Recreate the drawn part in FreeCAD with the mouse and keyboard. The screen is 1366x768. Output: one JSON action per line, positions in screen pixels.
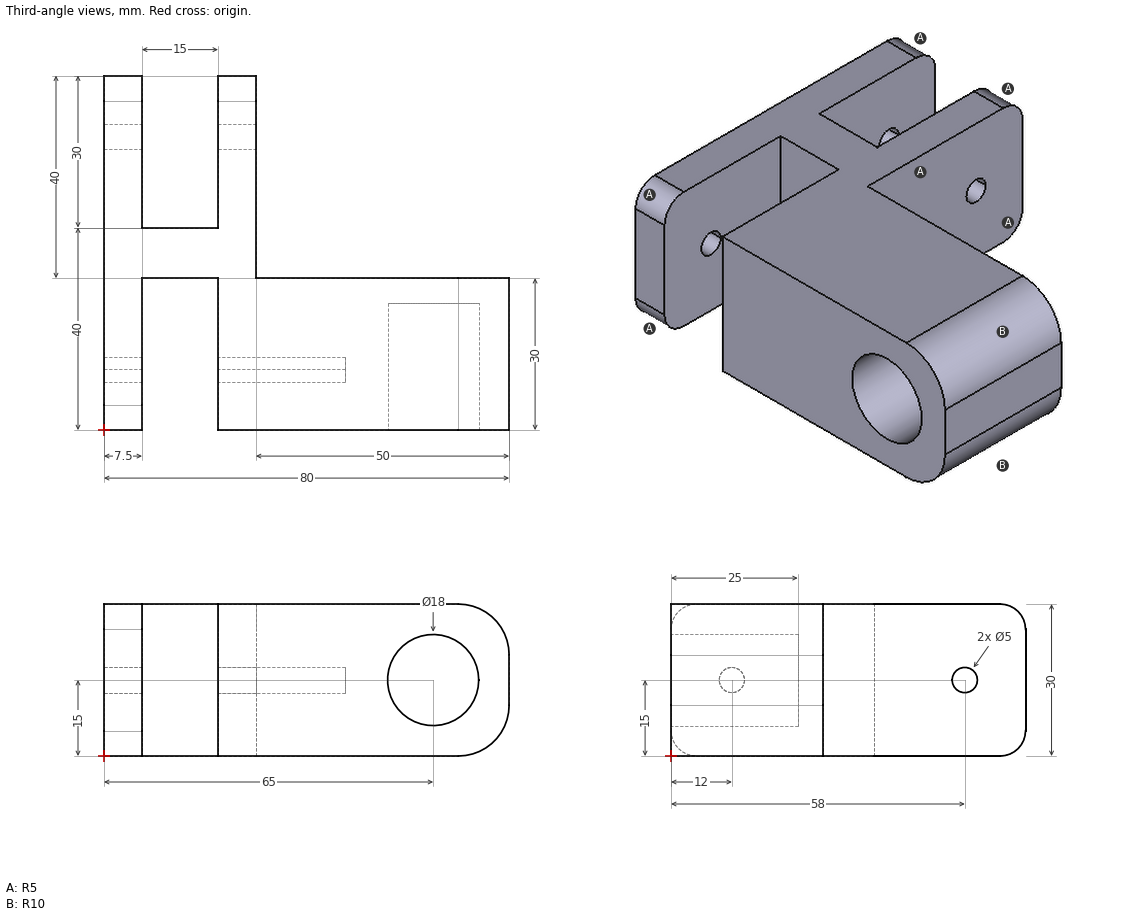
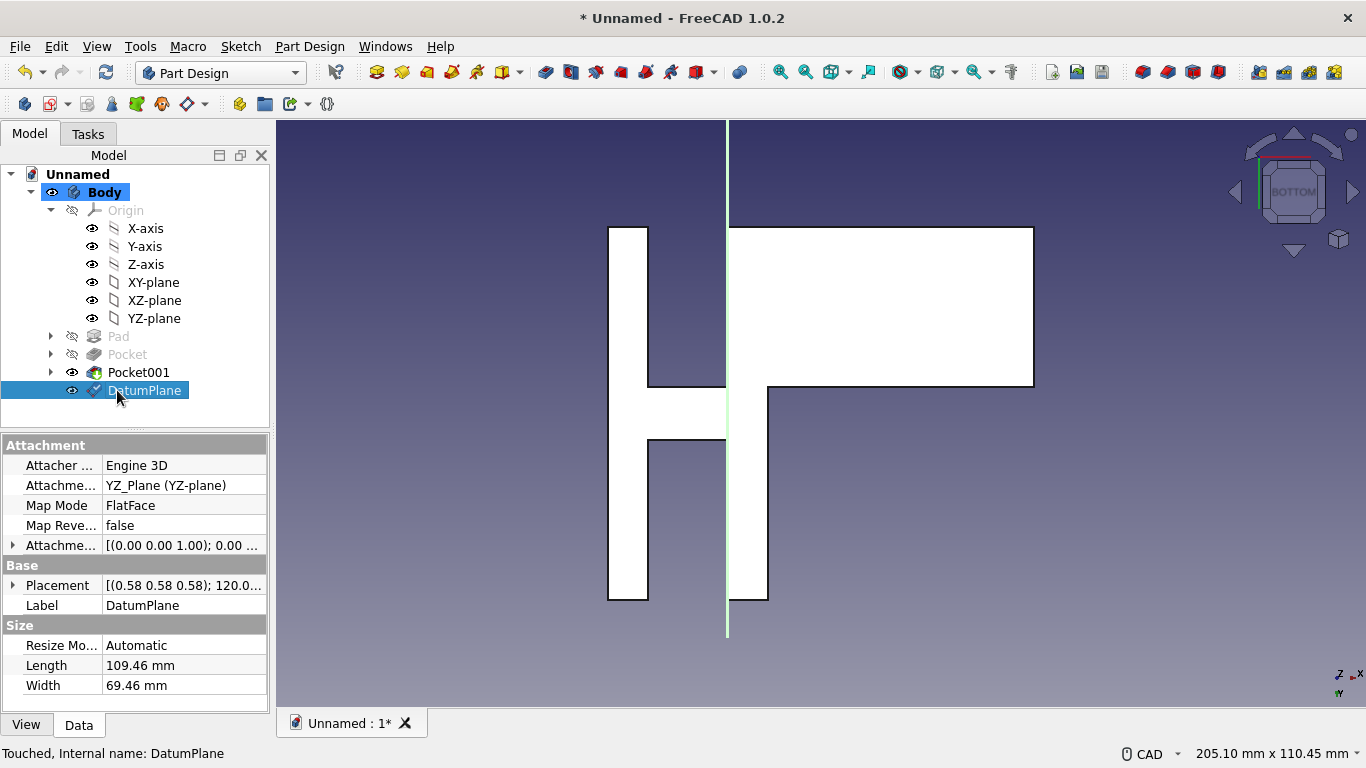
{"action": "left_click", "coordinate": [50, 104]}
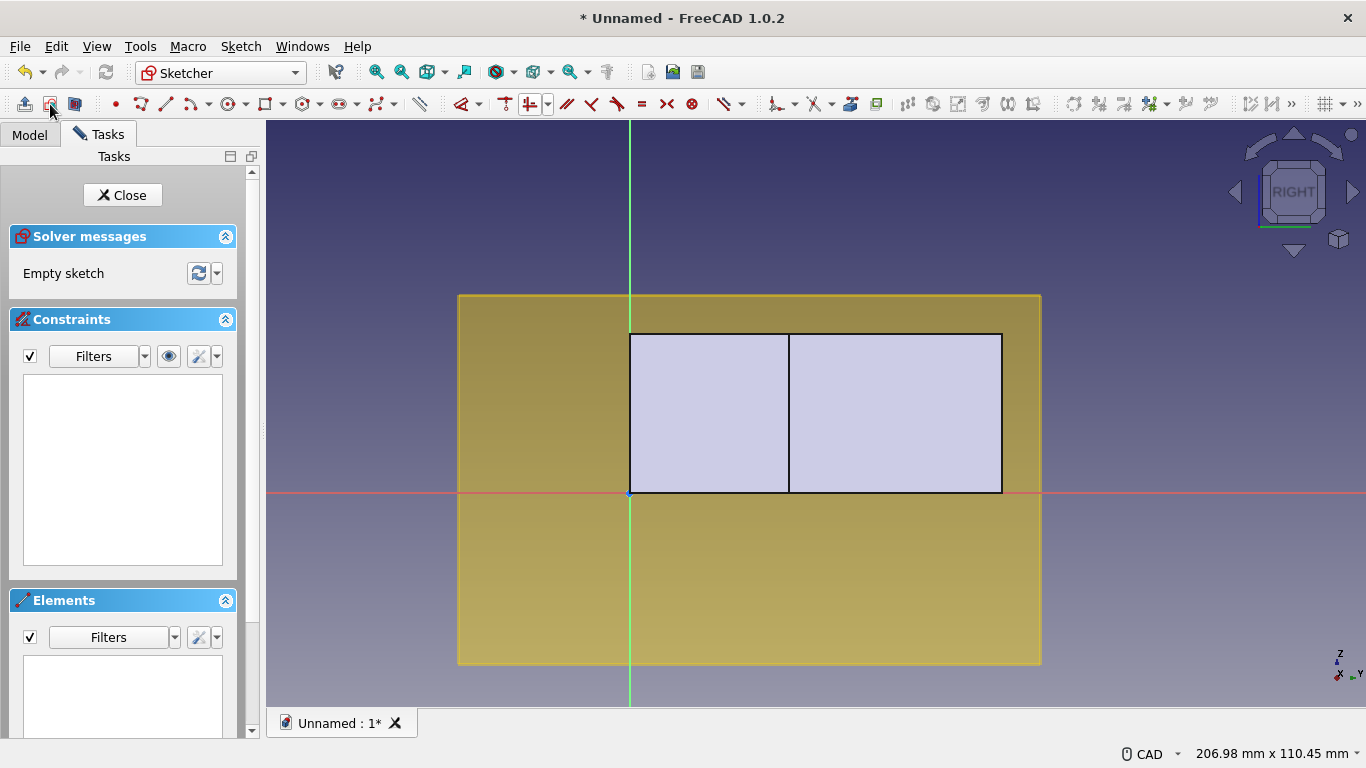
{"action": "key", "text": "q s"}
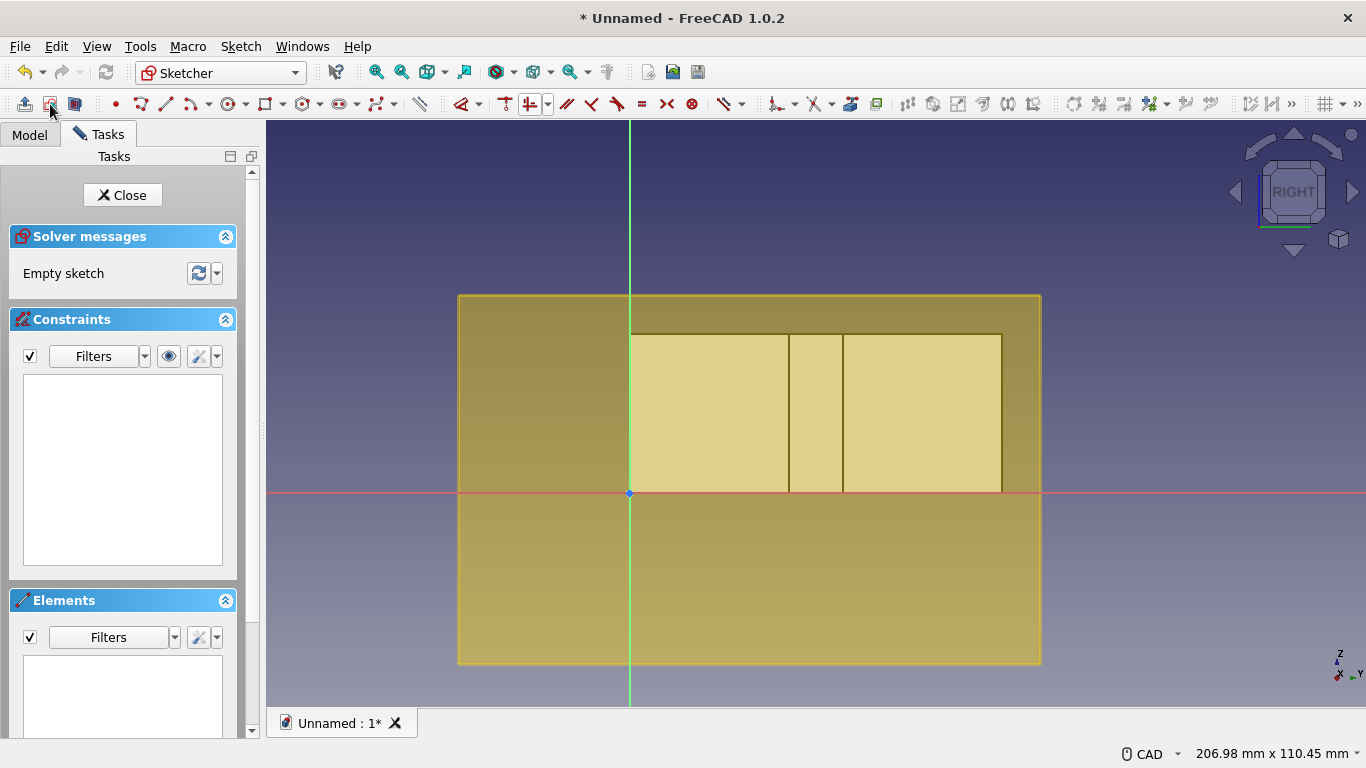
{"action": "scroll", "coordinate": [843, 487], "scroll_direction": "up", "scroll_amount": 3}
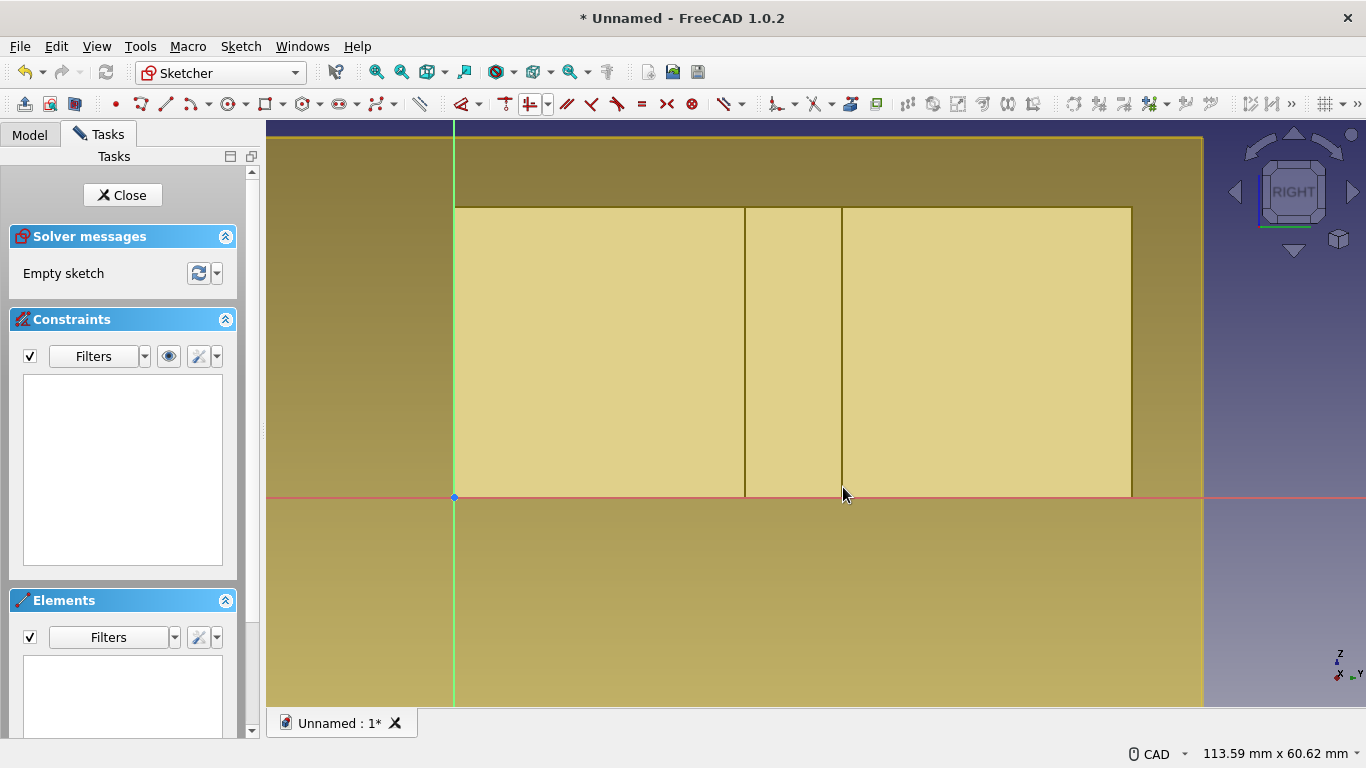
{"action": "left_click", "coordinate": [228, 104]}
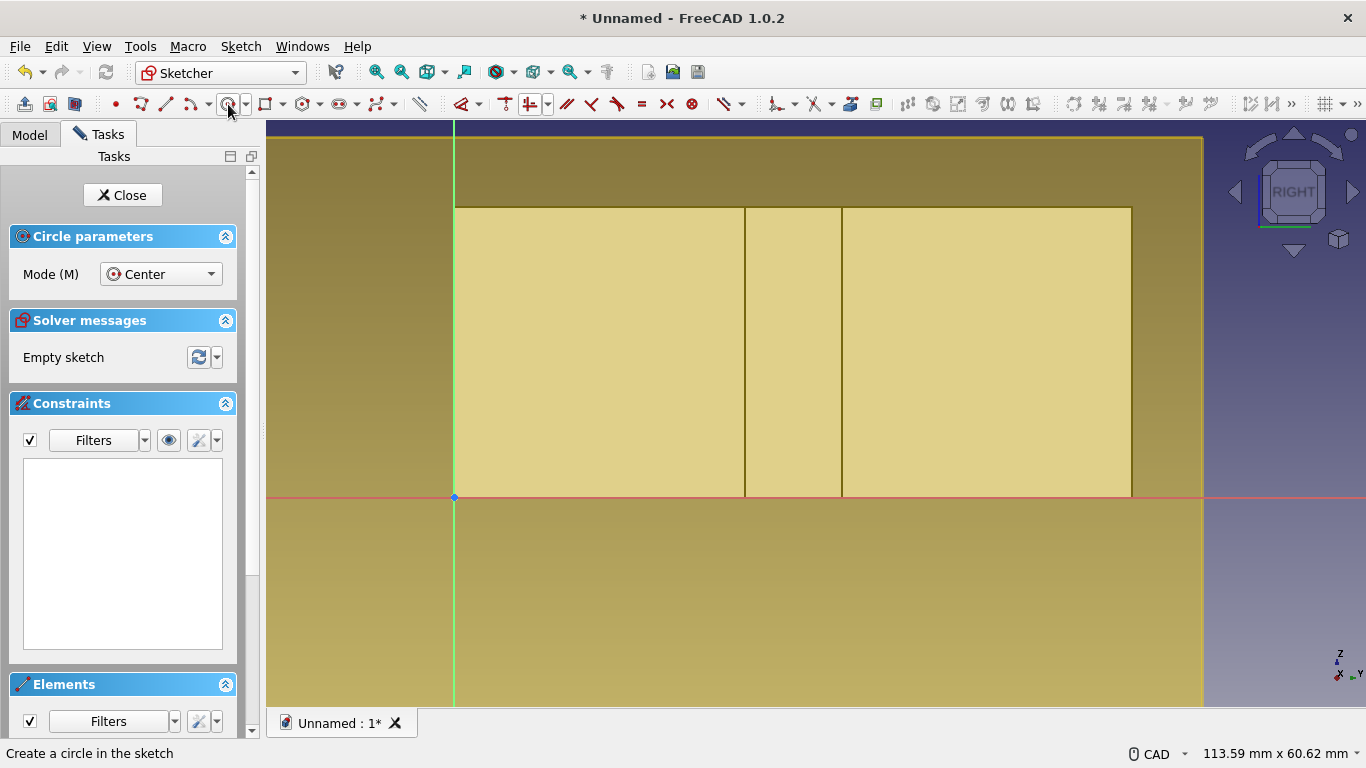
{"action": "left_click", "coordinate": [1016, 353]}
{"action": "left_click", "coordinate": [1033, 335]}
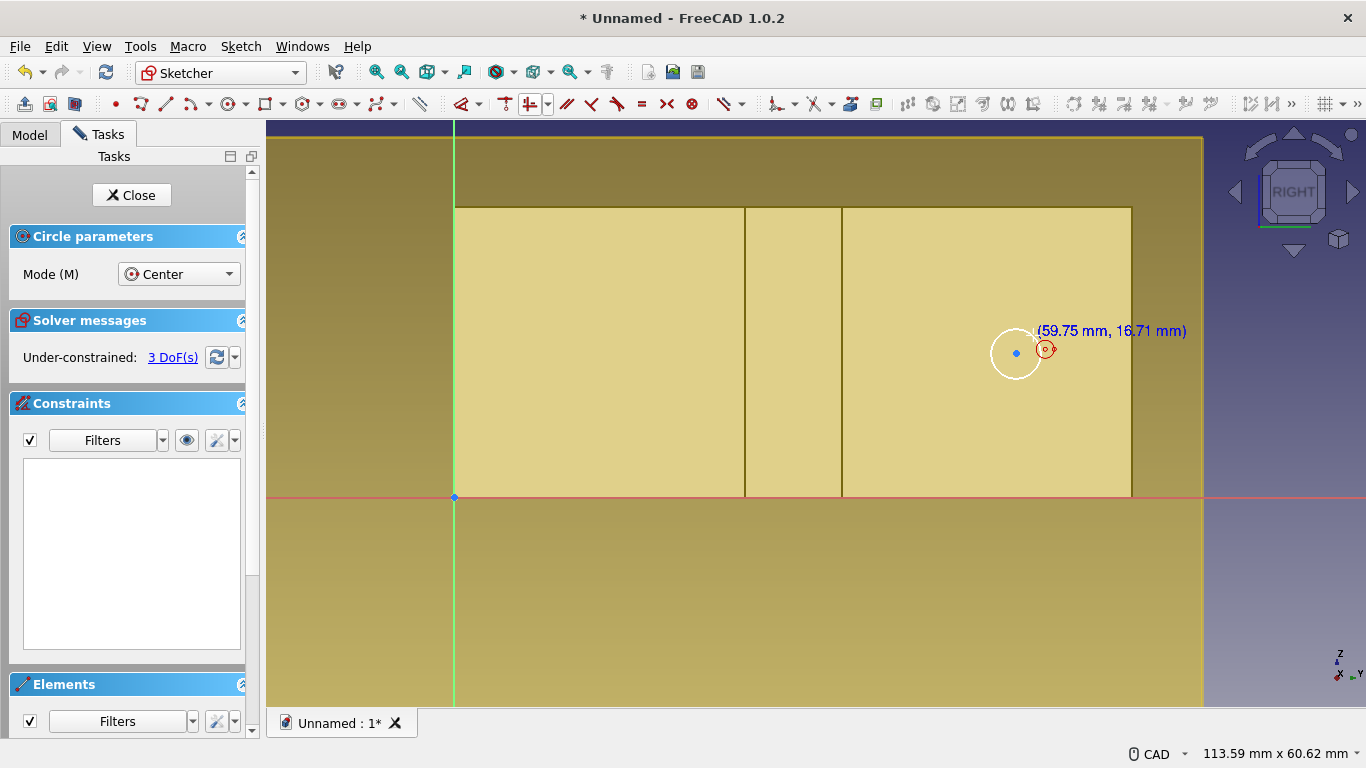
{"action": "left_click", "coordinate": [571, 353]}
{"action": "left_click", "coordinate": [588, 335]}
{"action": "key", "text": "Escape"}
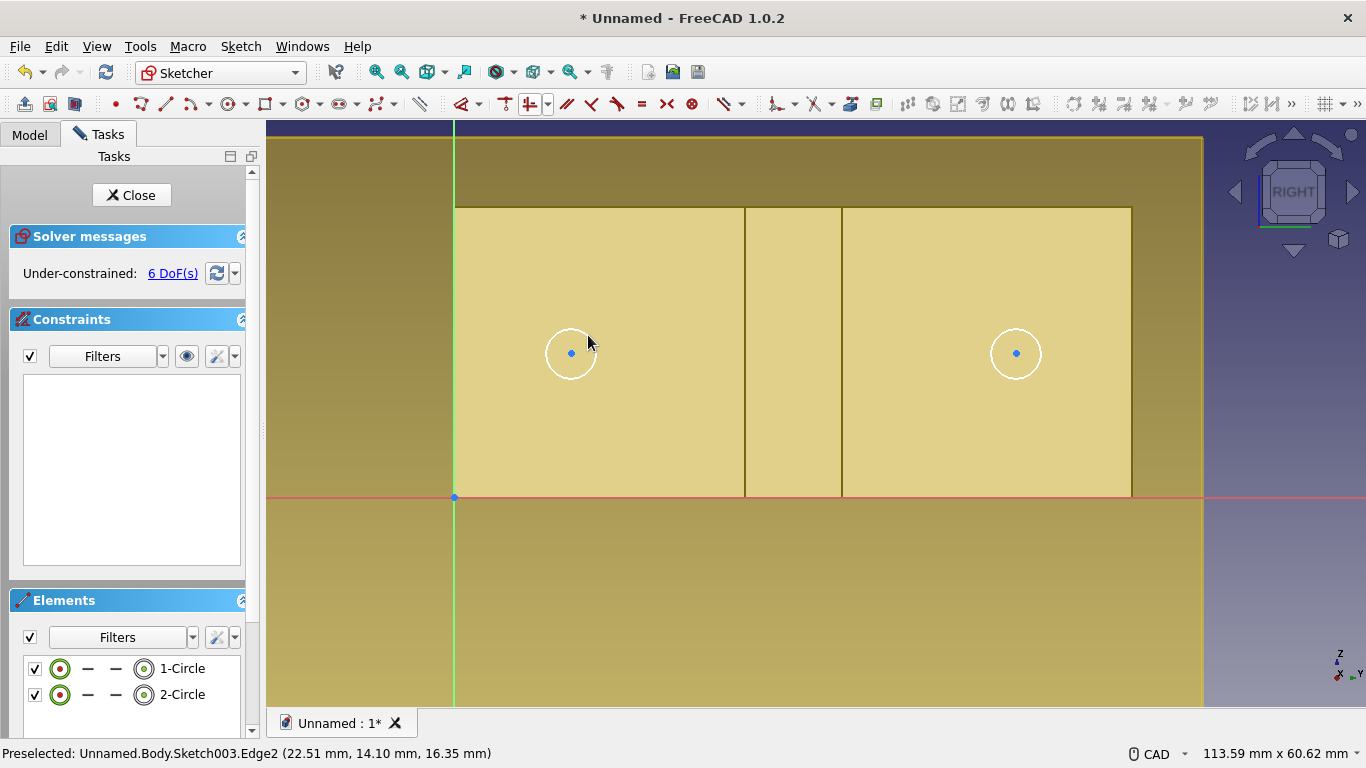
{"action": "left_click", "coordinate": [1033, 336]}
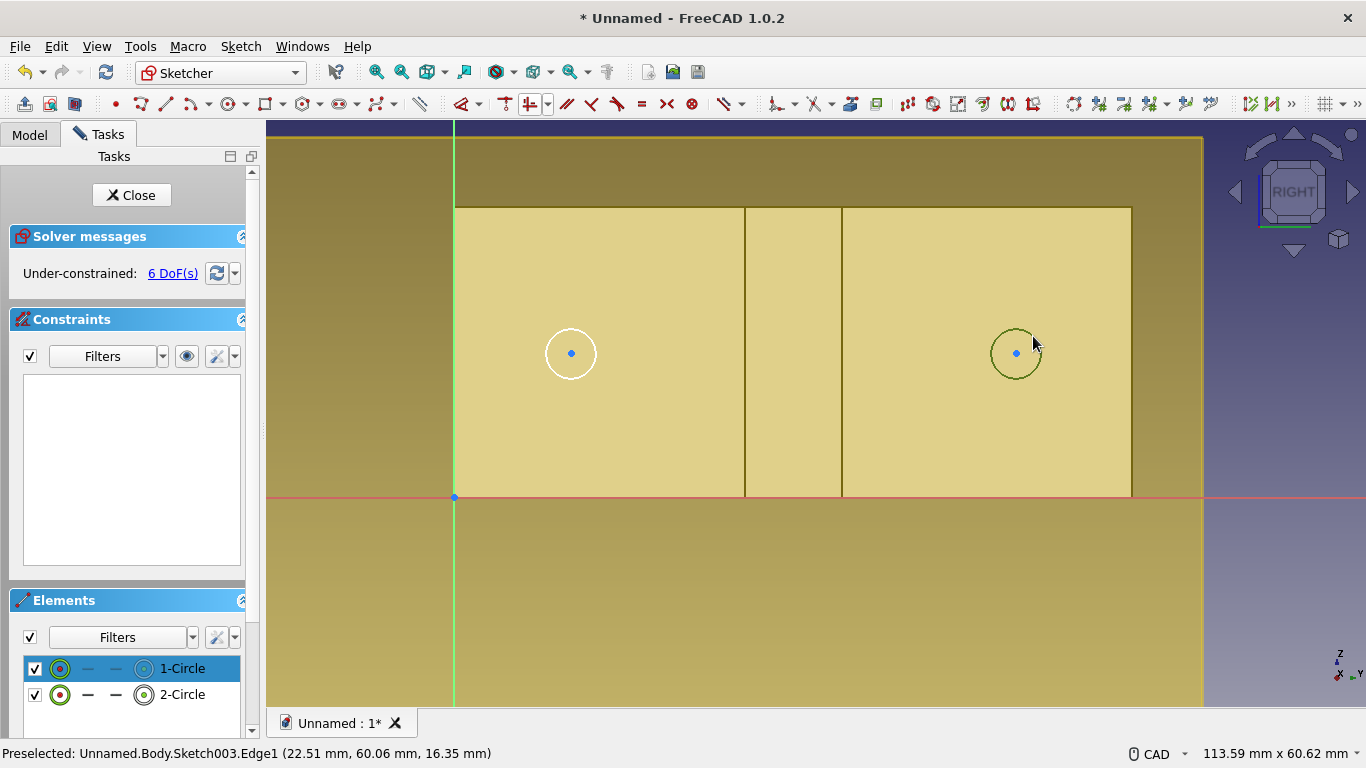
{"action": "left_click", "coordinate": [588, 336]}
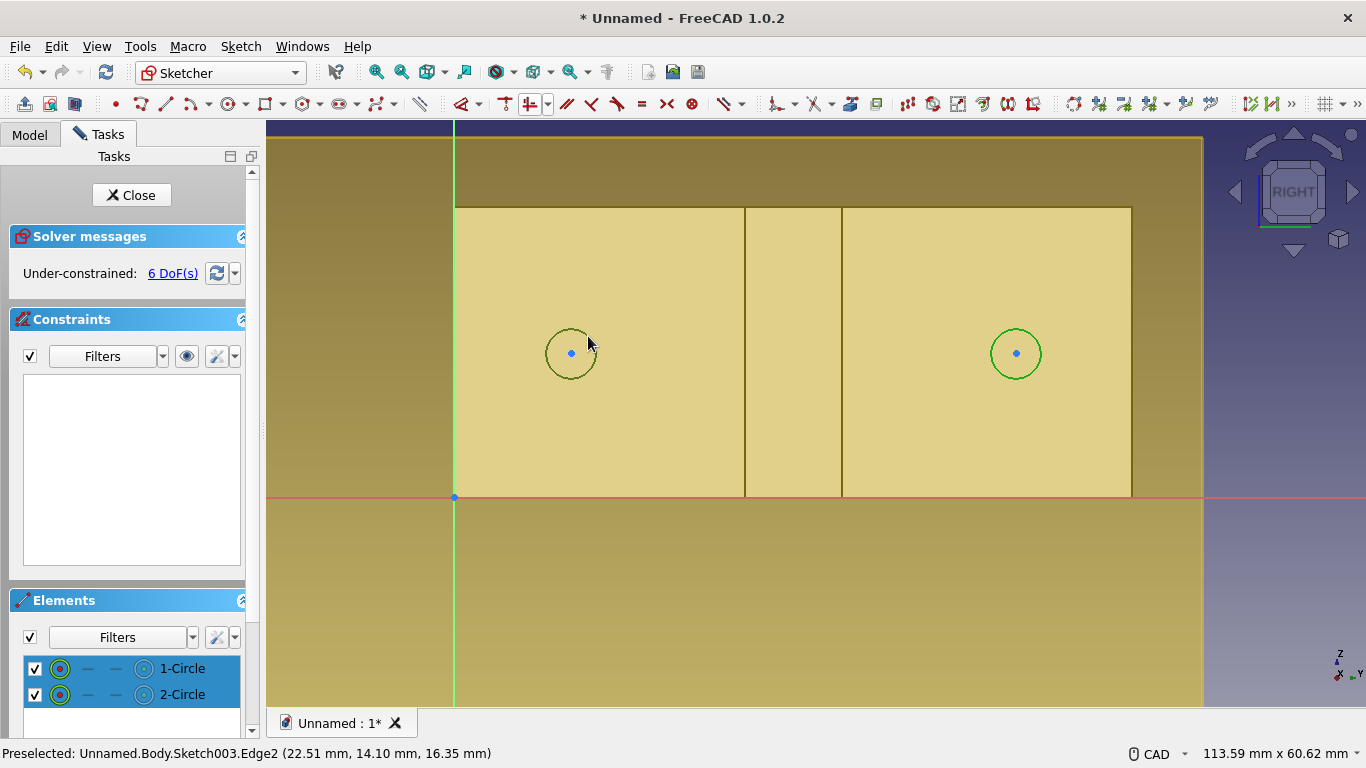
{"action": "key", "text": "e"}